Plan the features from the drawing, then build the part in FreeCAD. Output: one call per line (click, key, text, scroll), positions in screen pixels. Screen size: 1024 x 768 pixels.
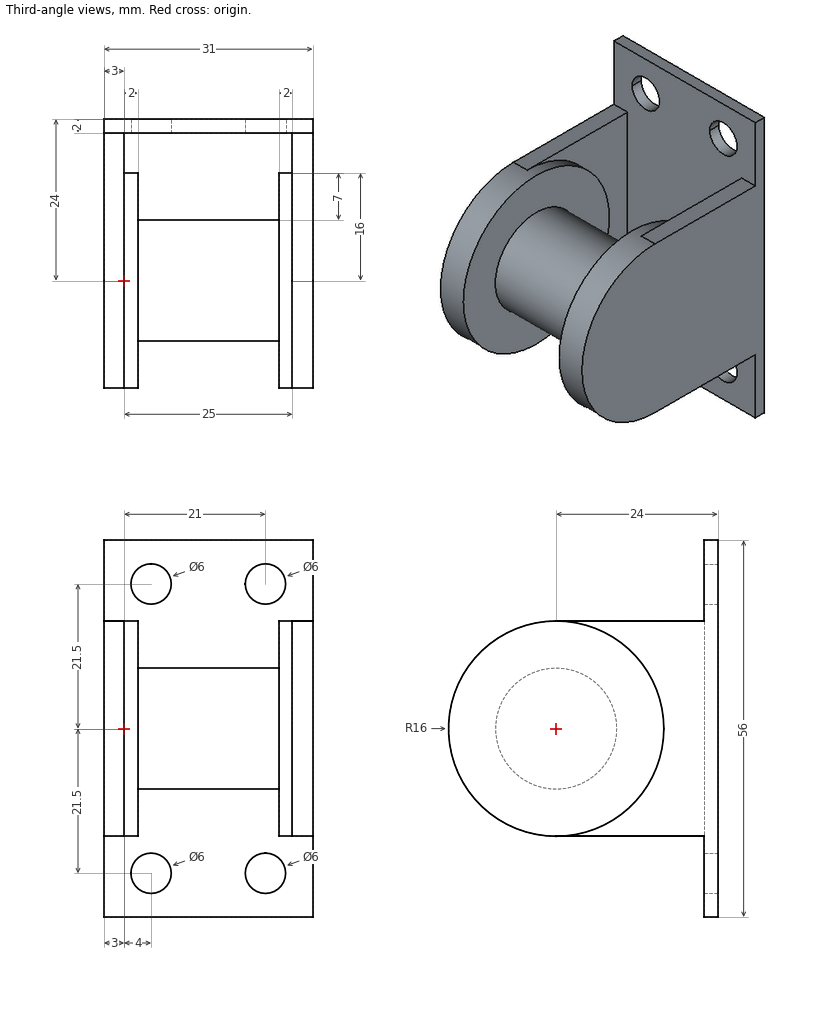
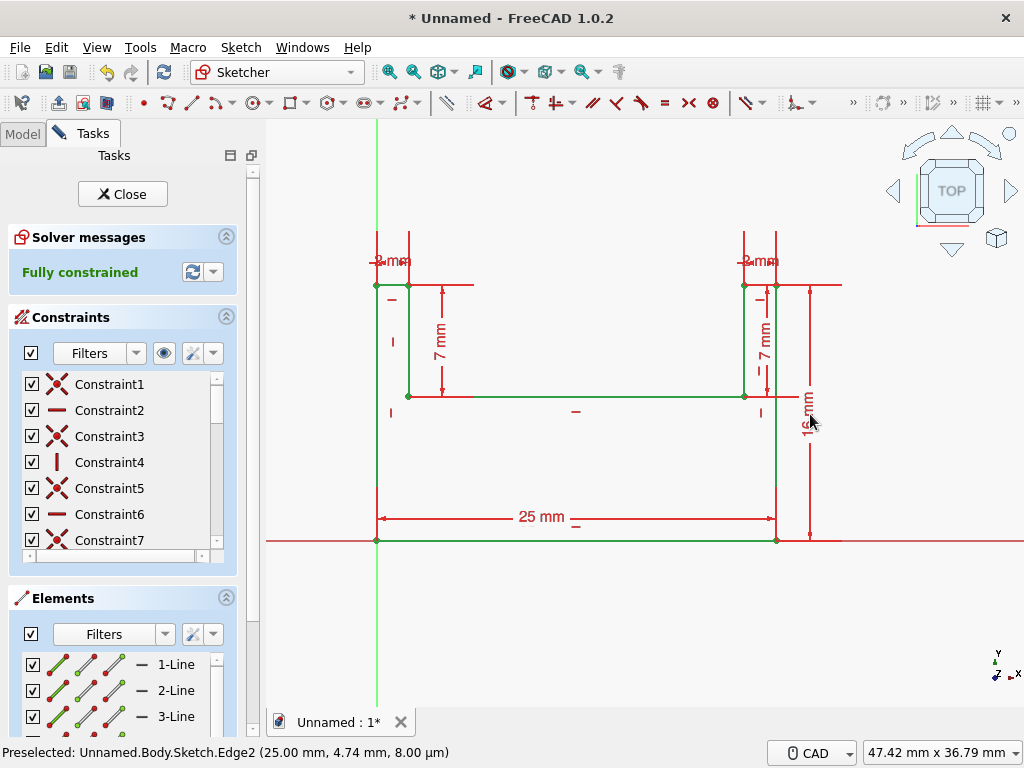
click(123, 194)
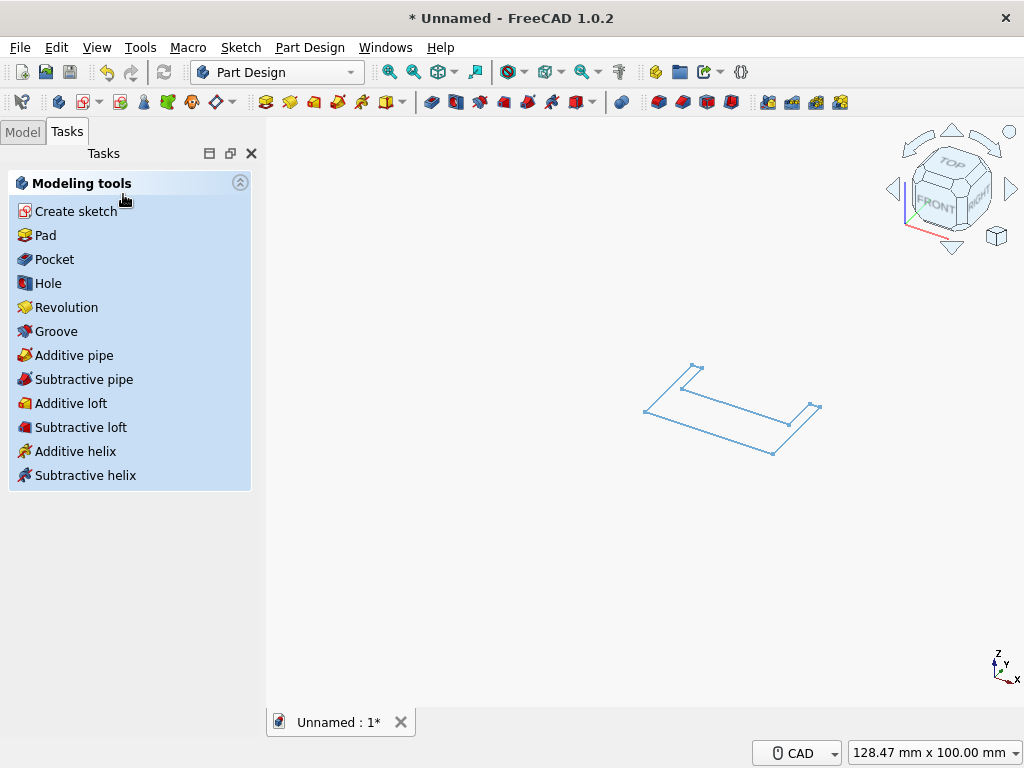
click(290, 102)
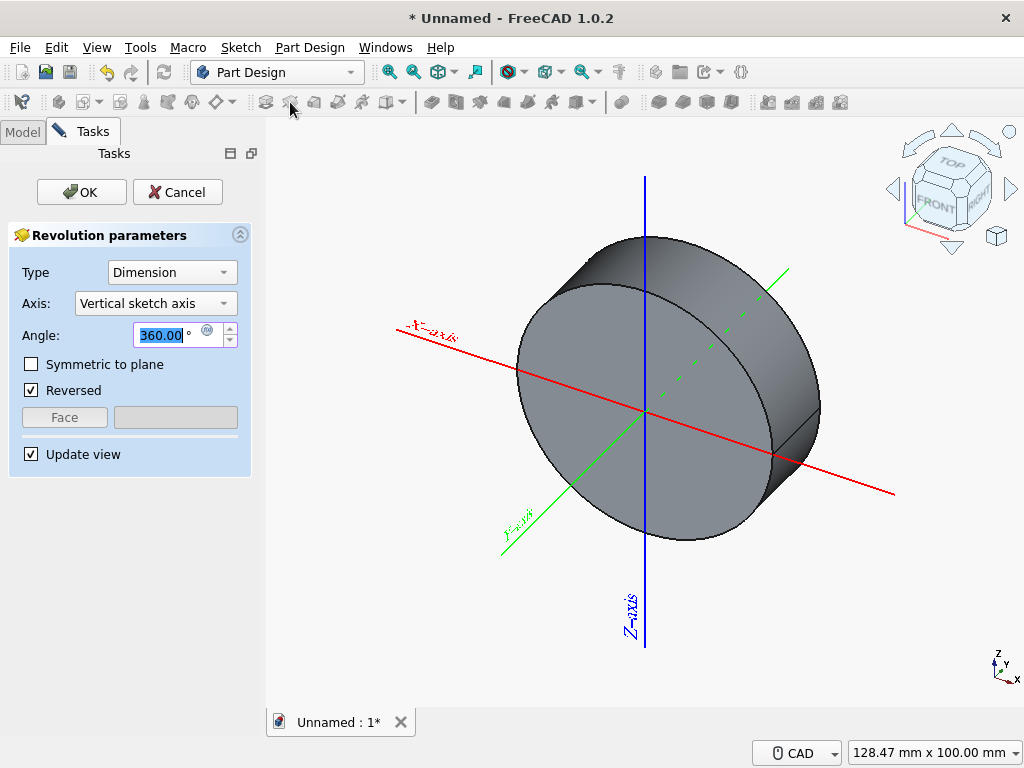
click(156, 304)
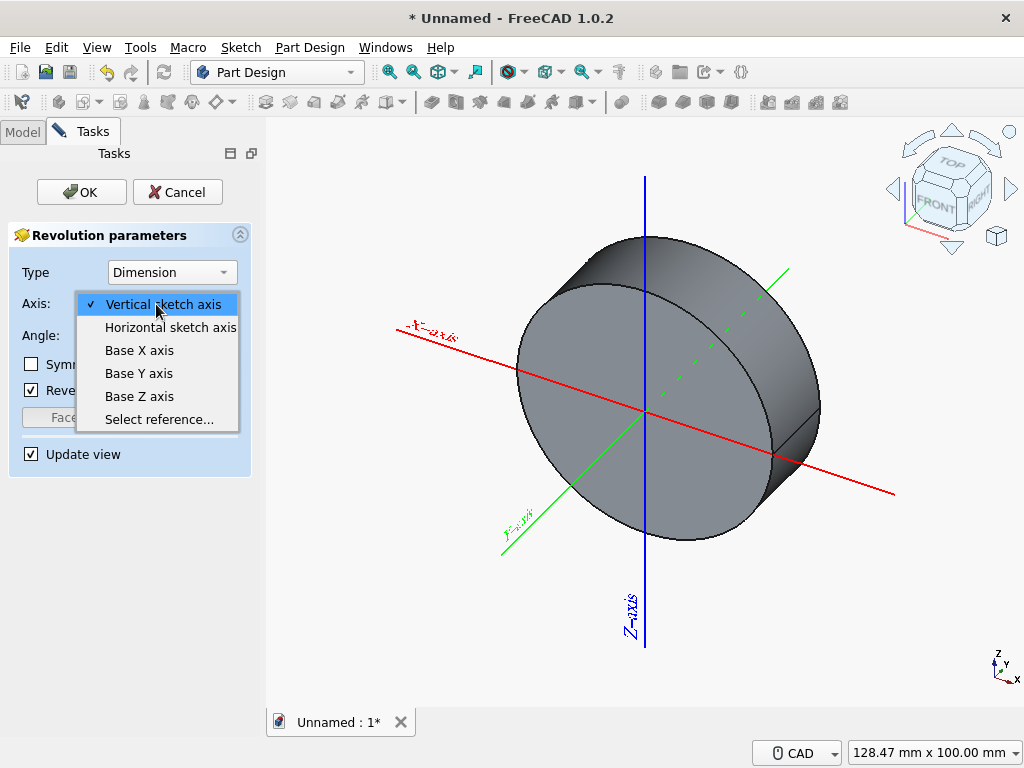
click(156, 328)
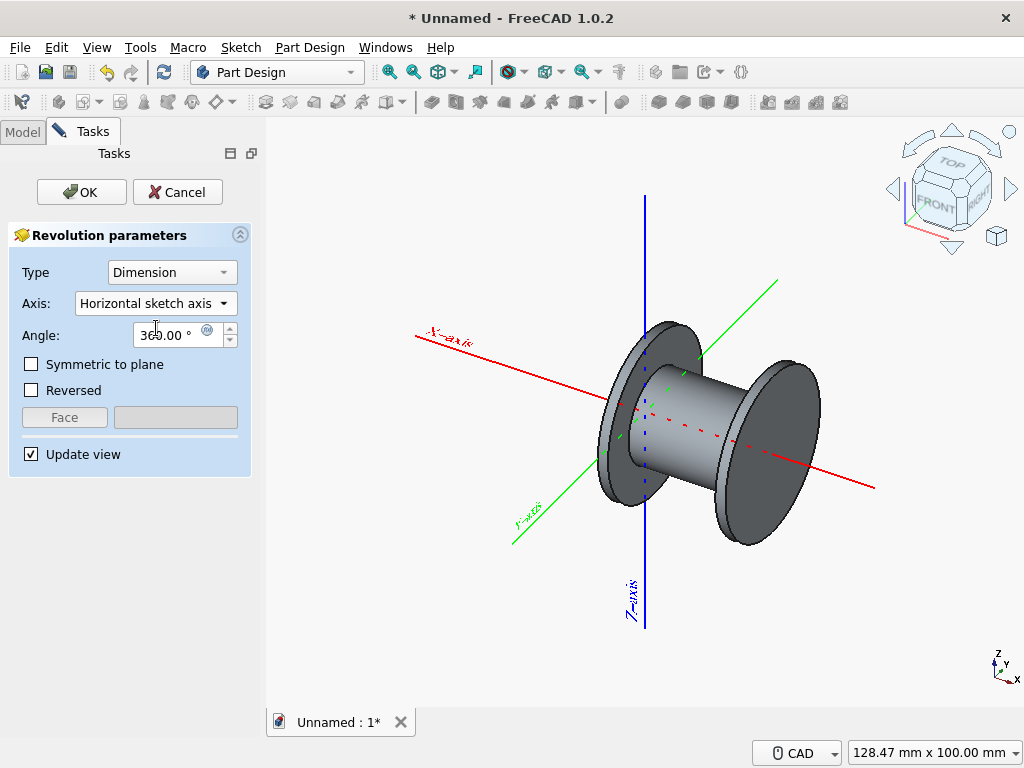
click(82, 192)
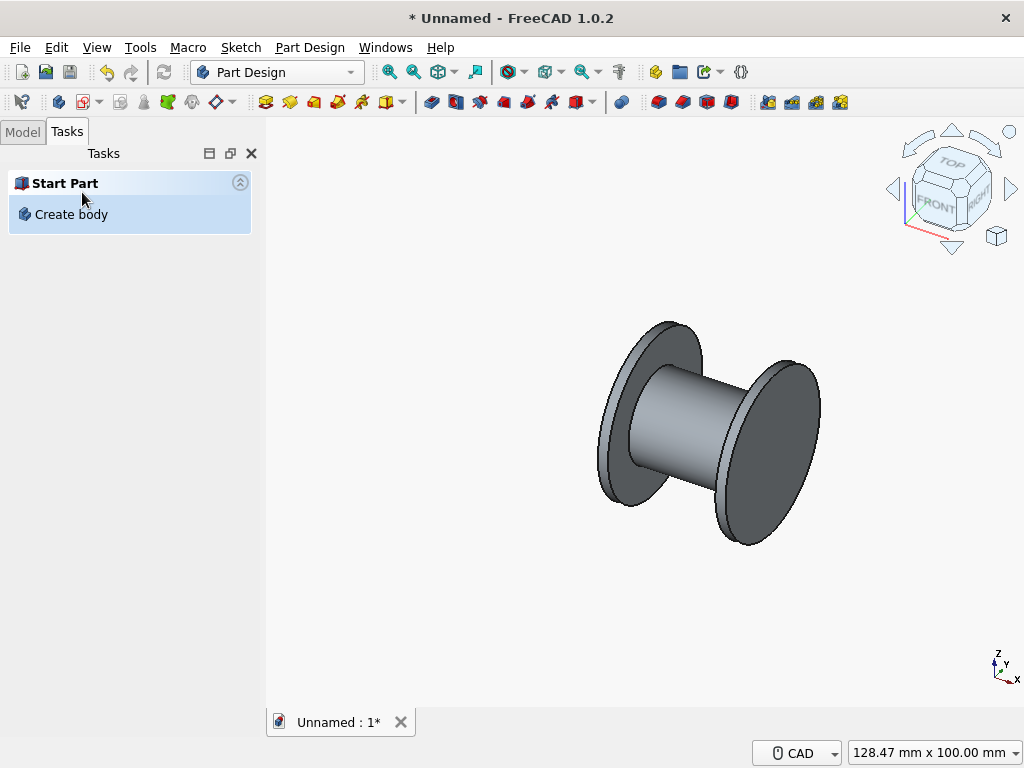
click(23, 131)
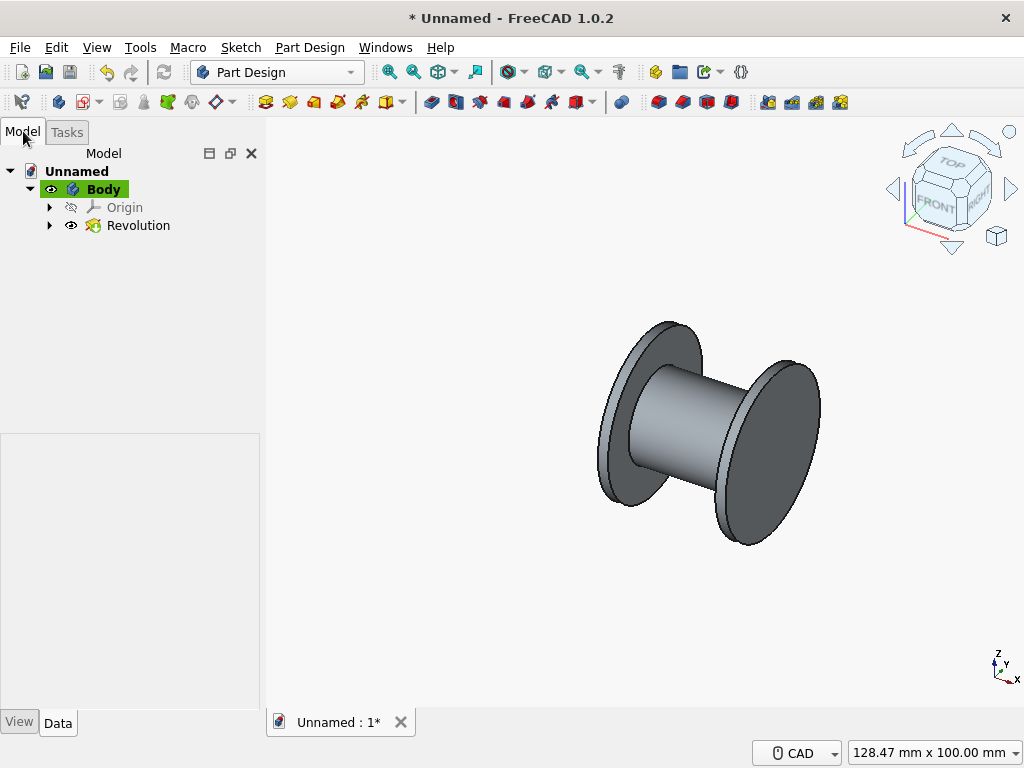
click(50, 207)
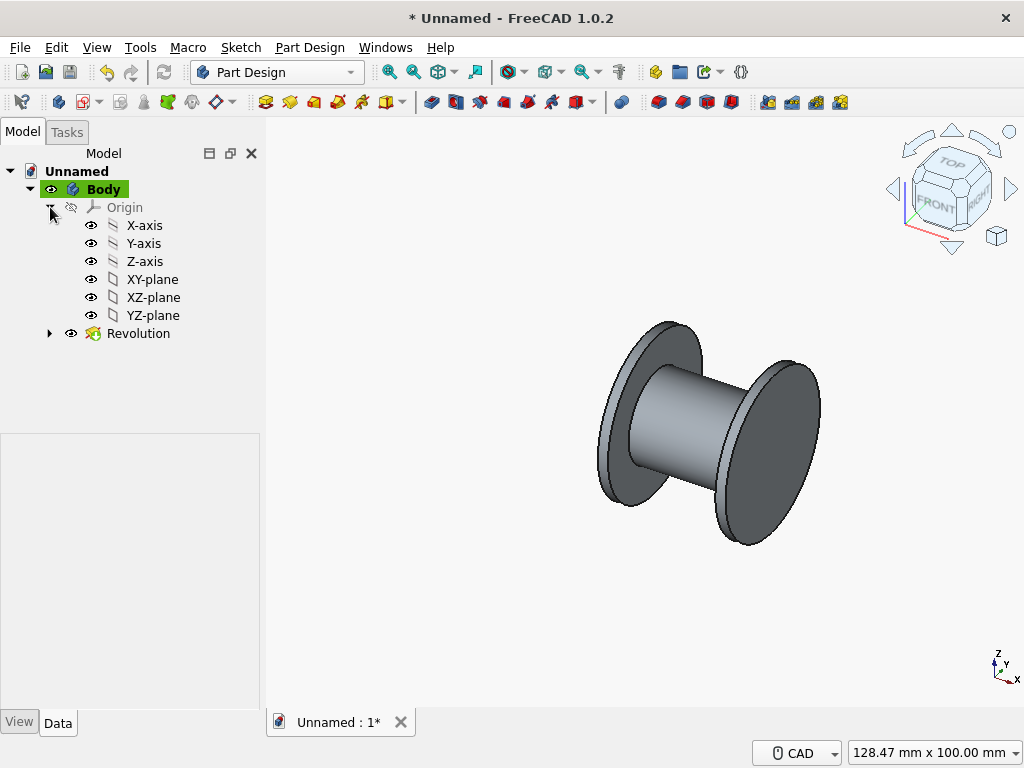
click(136, 315)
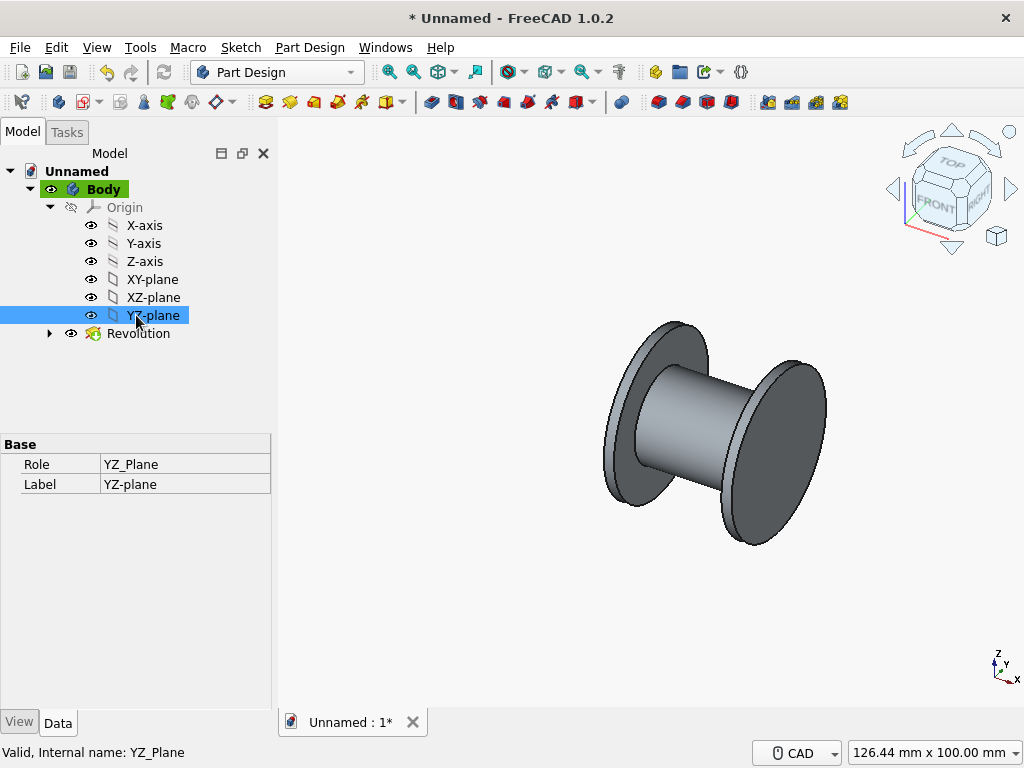
click(216, 102)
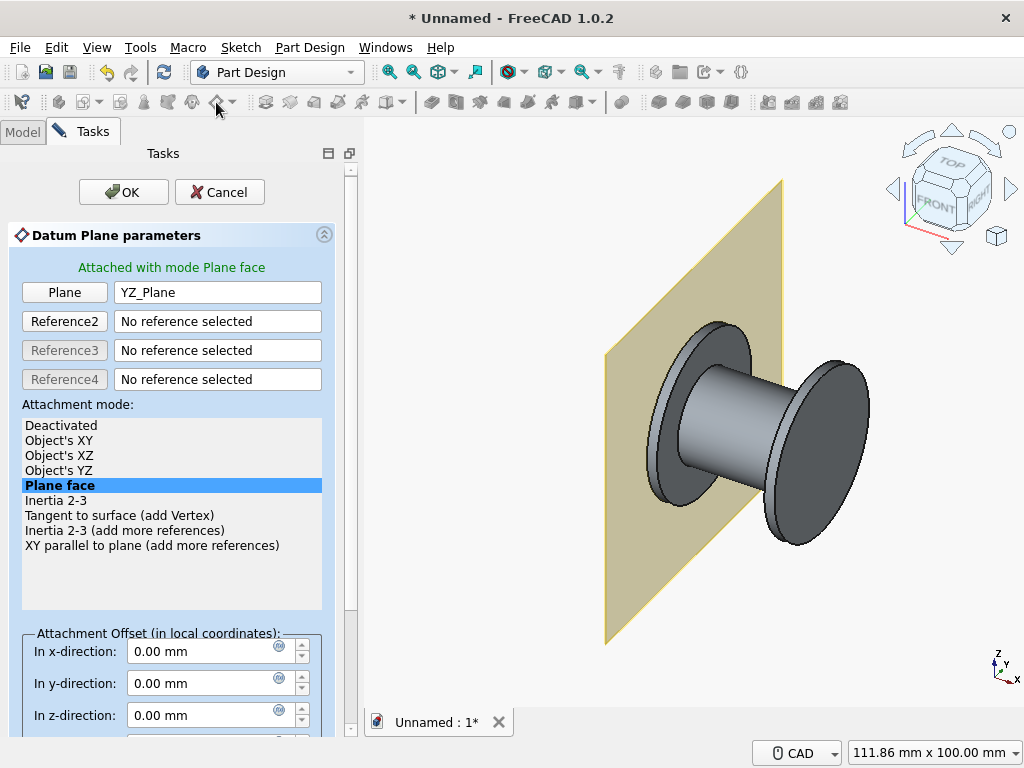
triple_click(210, 715)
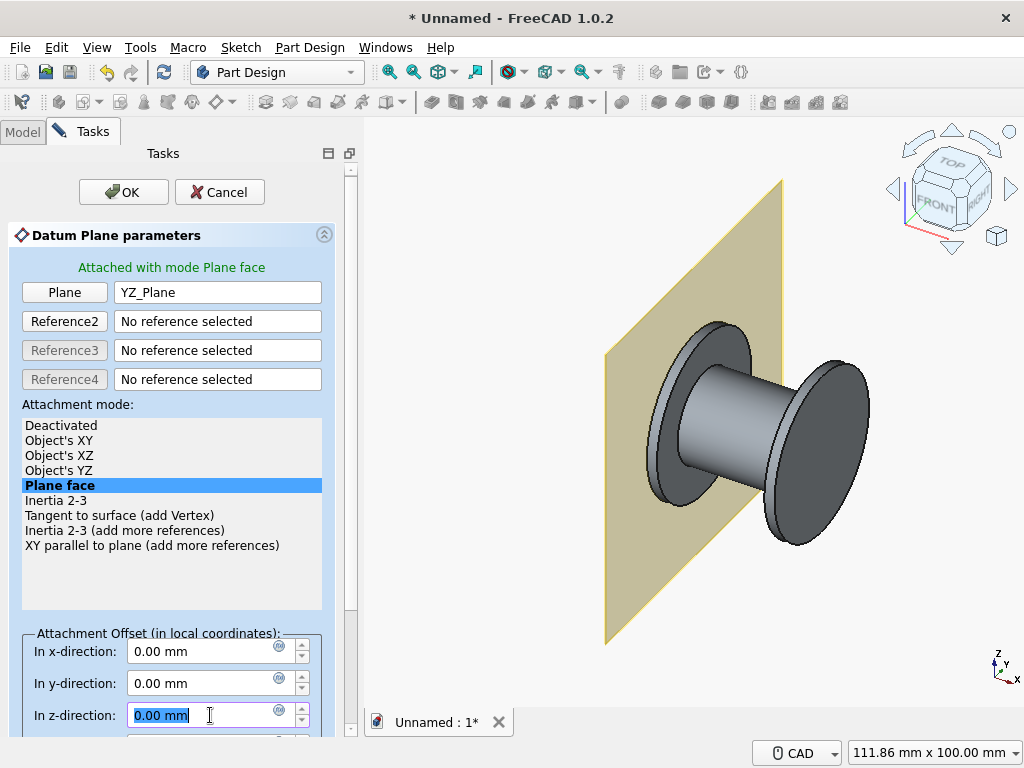
text(-3)
key(Tab)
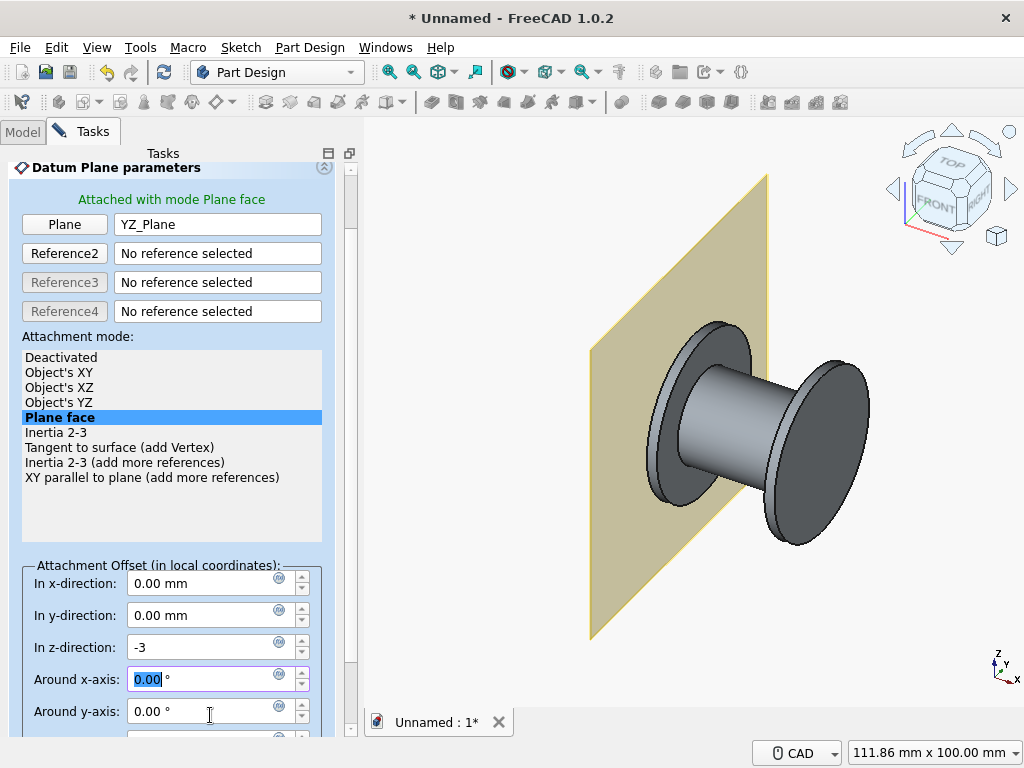
scroll(351, 450, up, 2)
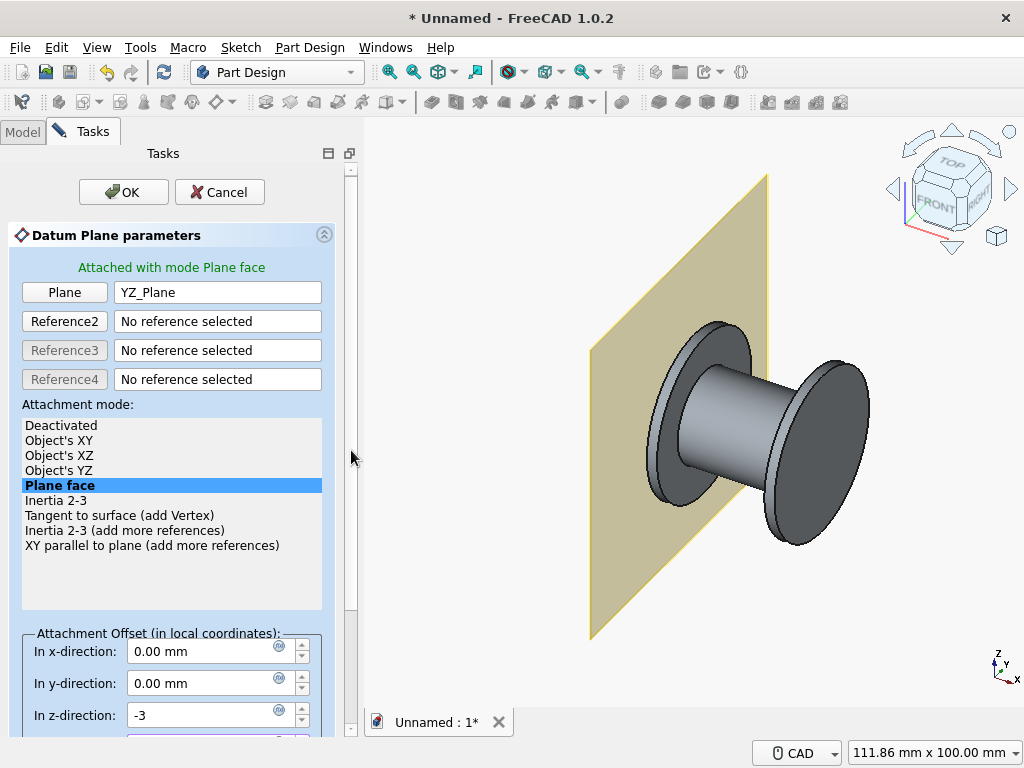
click(124, 192)